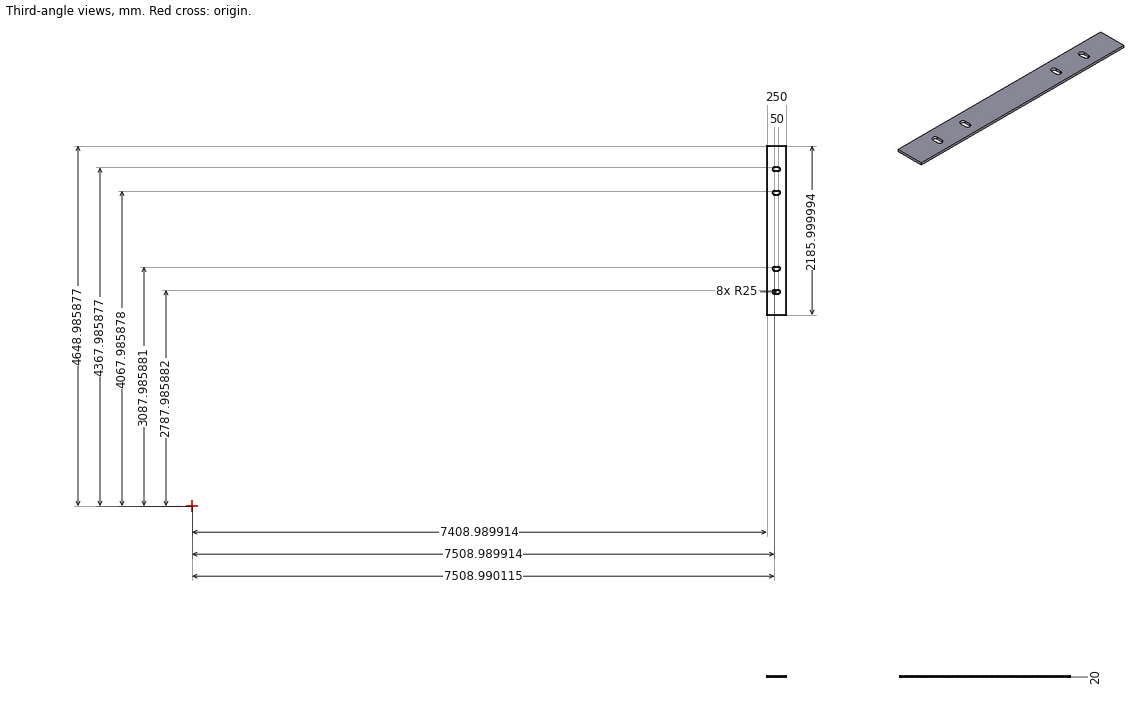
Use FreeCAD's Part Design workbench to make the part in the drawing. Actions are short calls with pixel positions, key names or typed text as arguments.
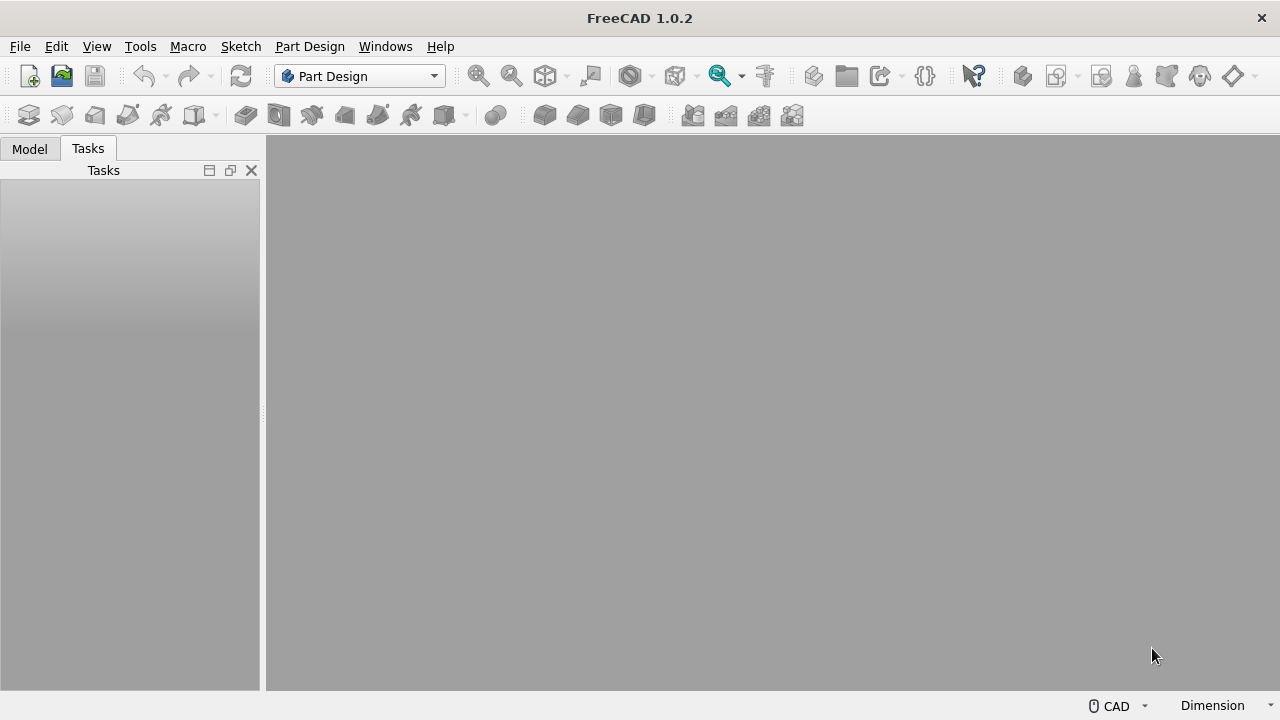
key(ctrl+n)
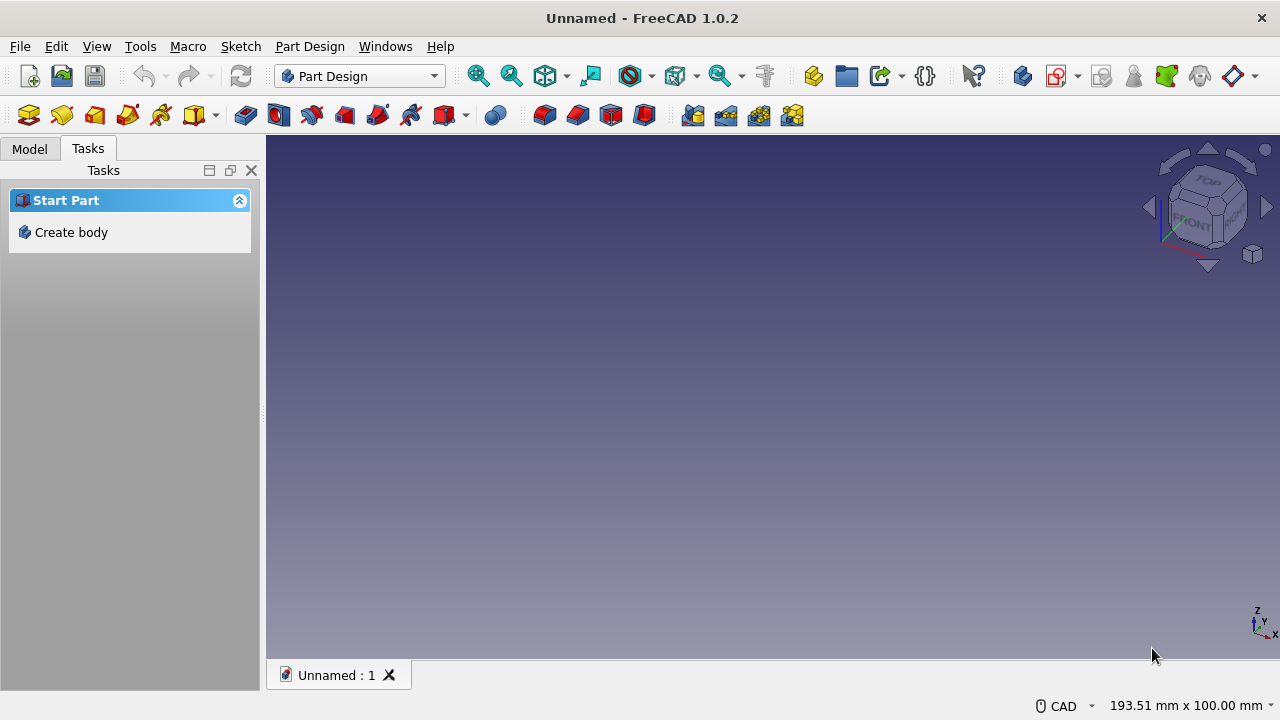
click(1056, 76)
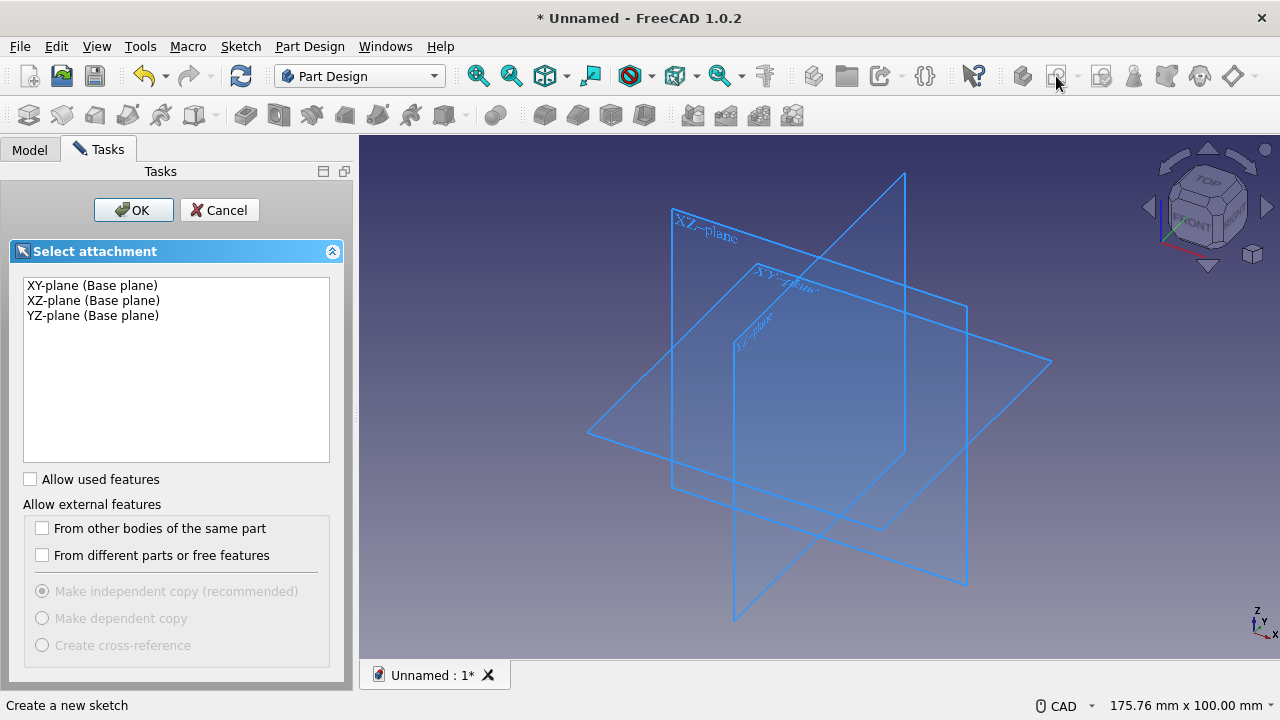
click(84, 286)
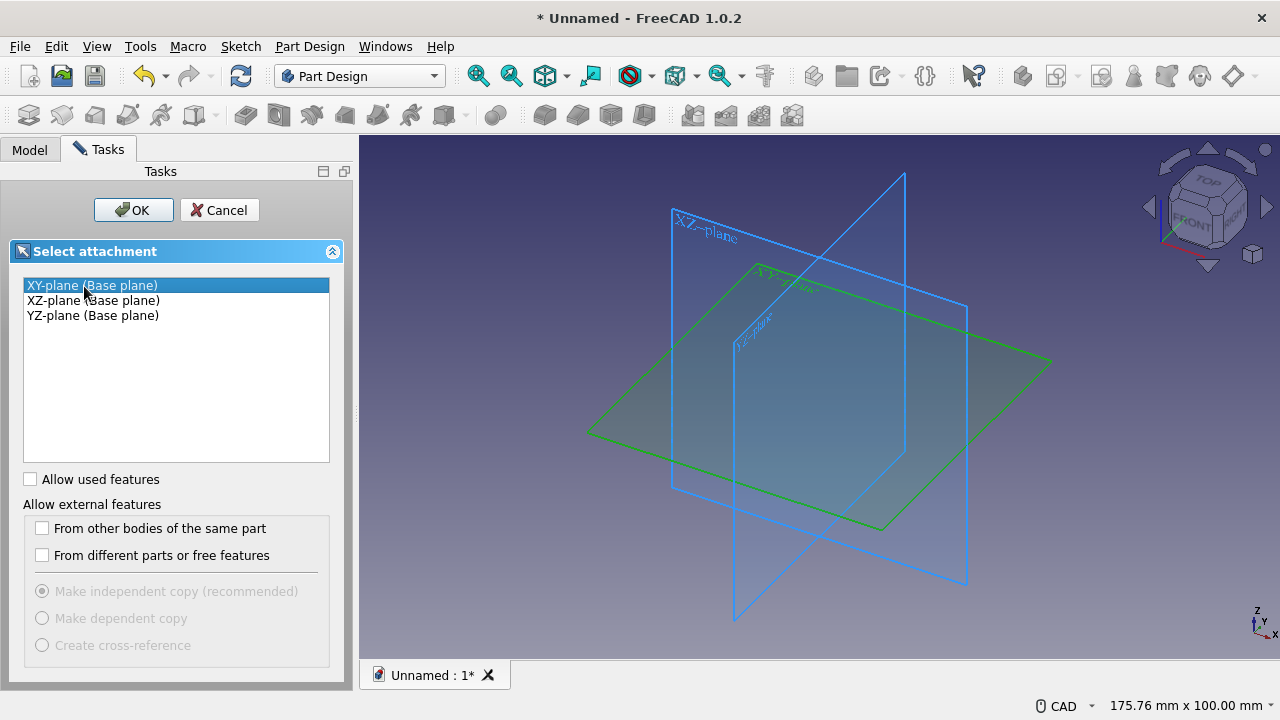
click(134, 210)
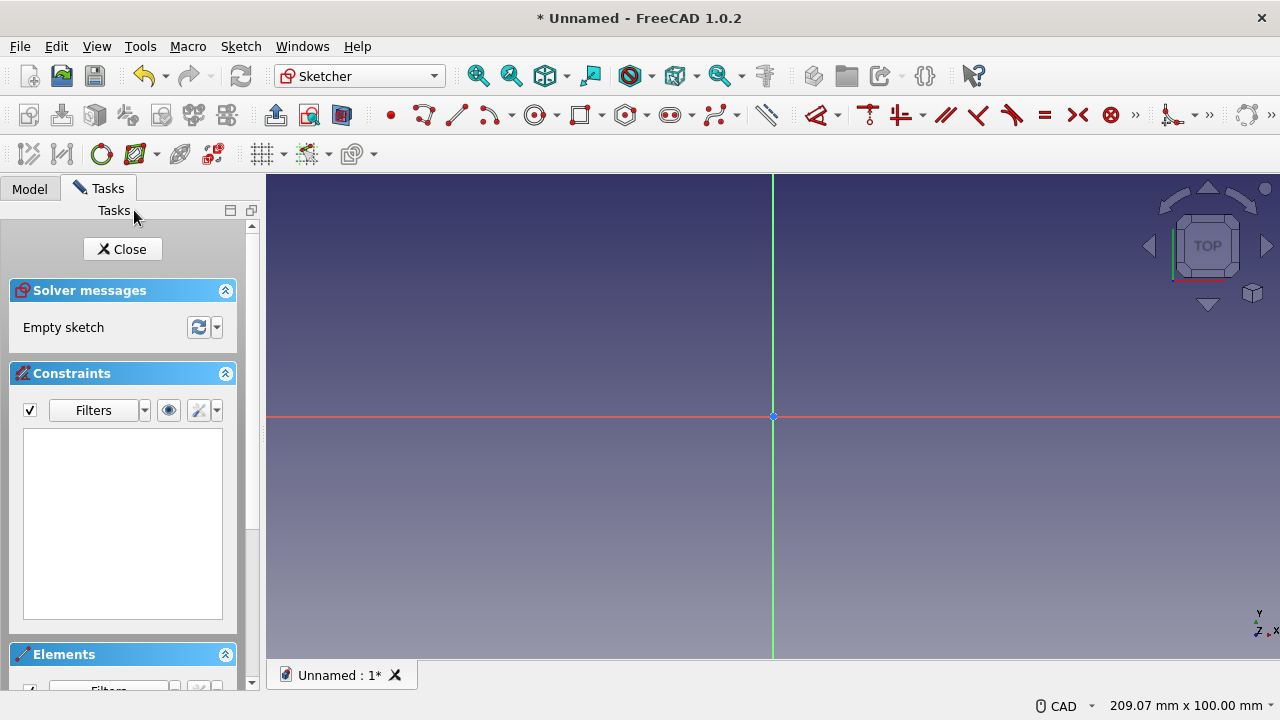
scroll(704, 416, down, 15)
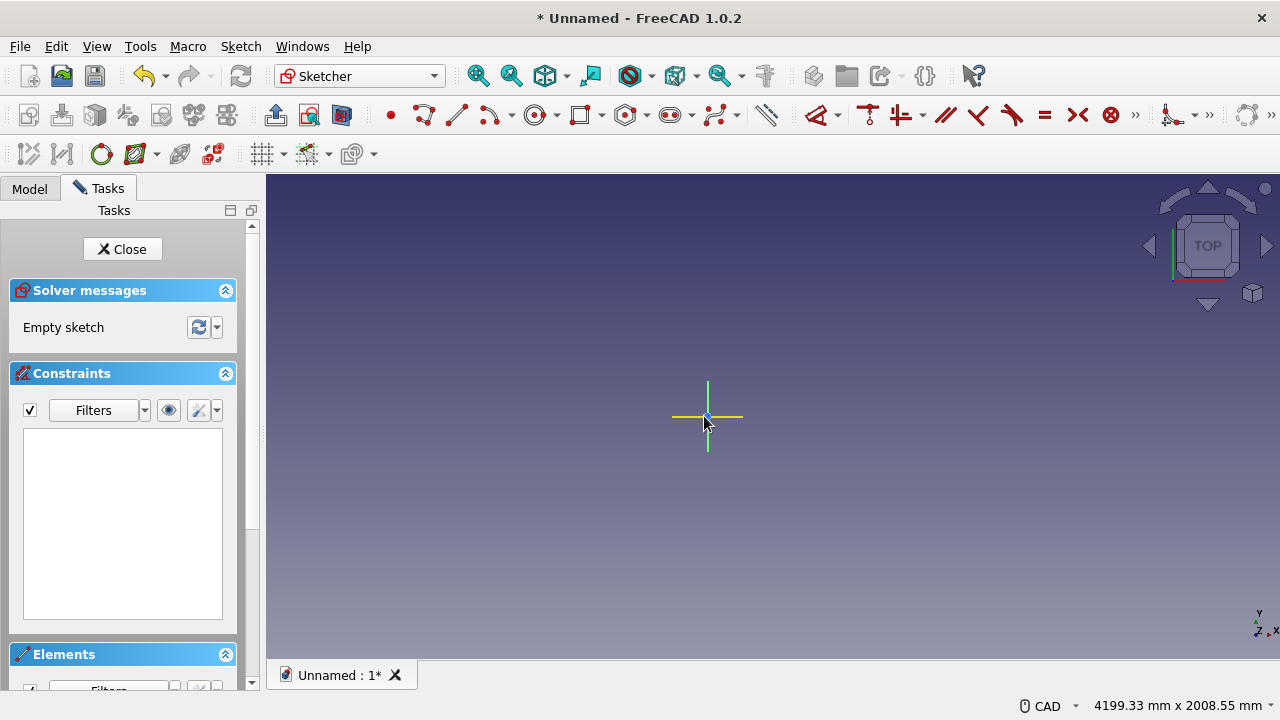
scroll(294, 631, down, 6)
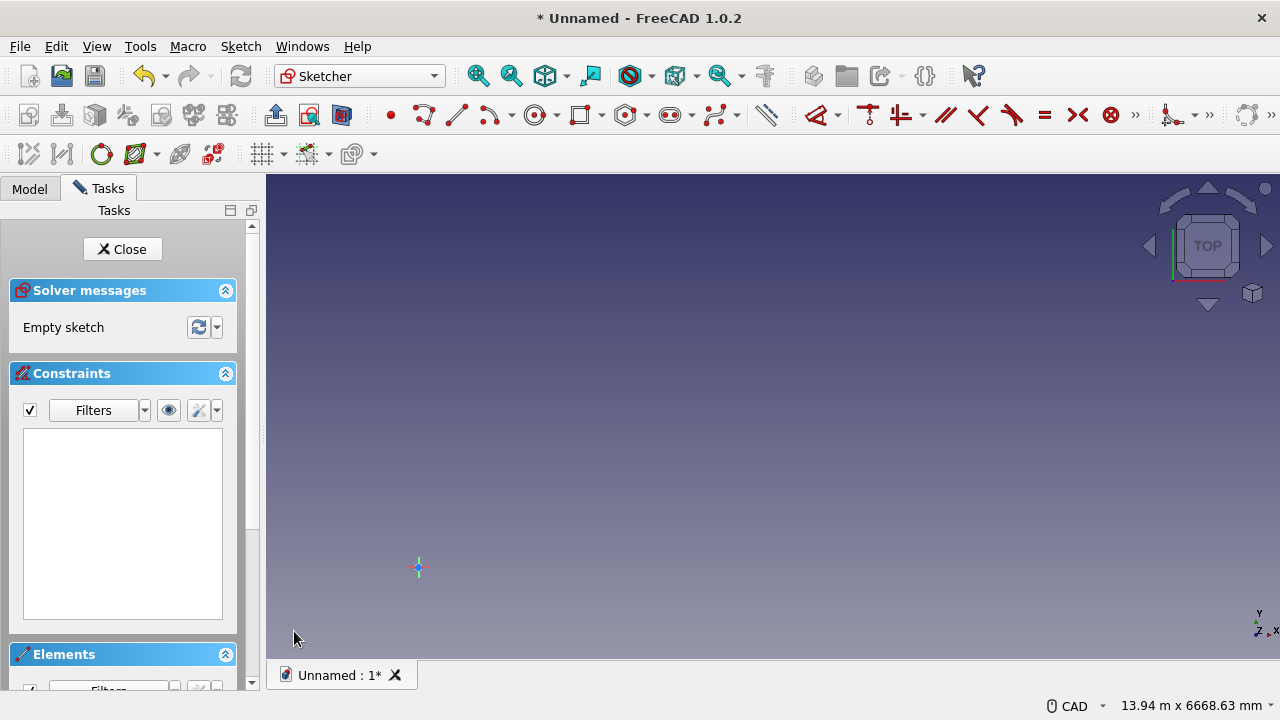
scroll(1115, 202, up, 3)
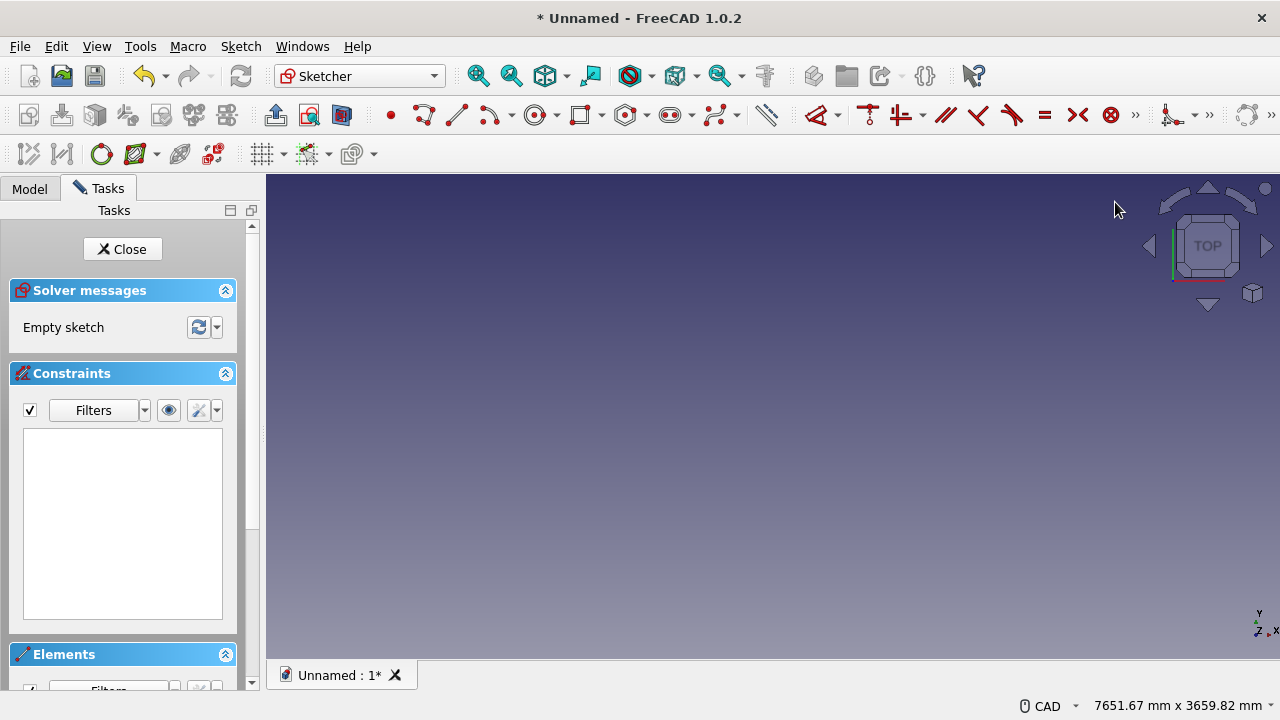
click(580, 116)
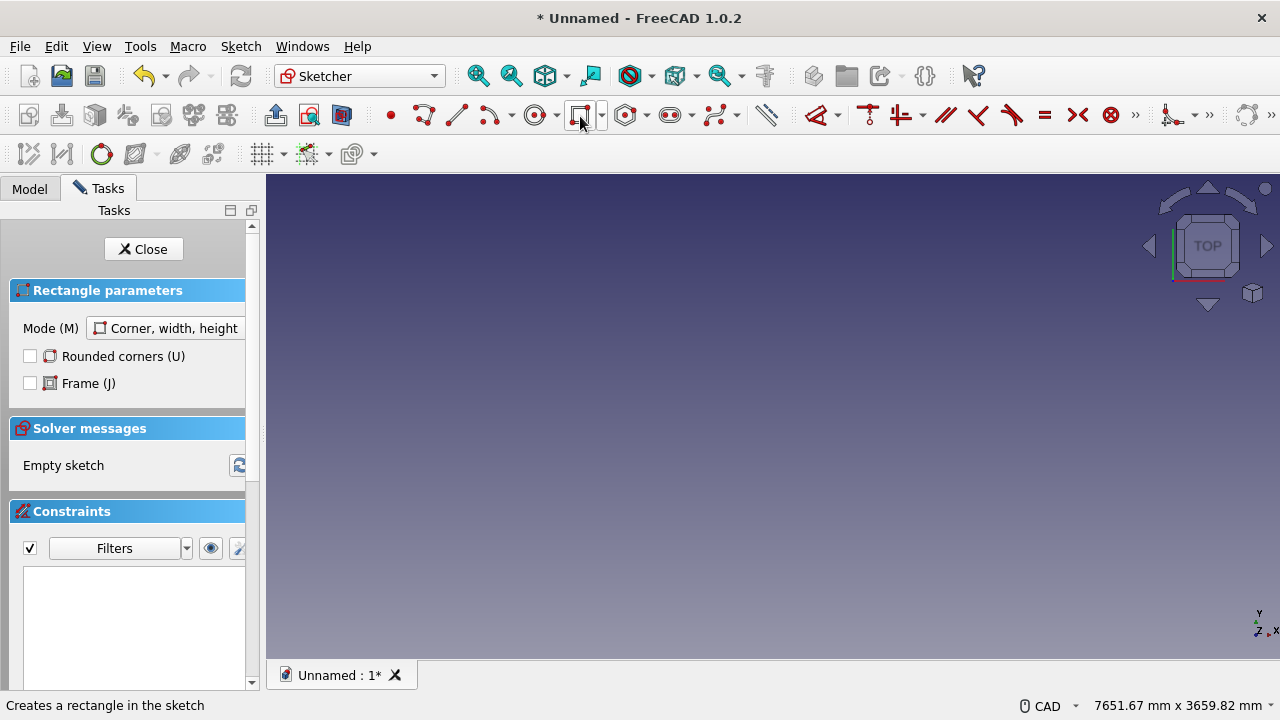
click(827, 251)
click(860, 541)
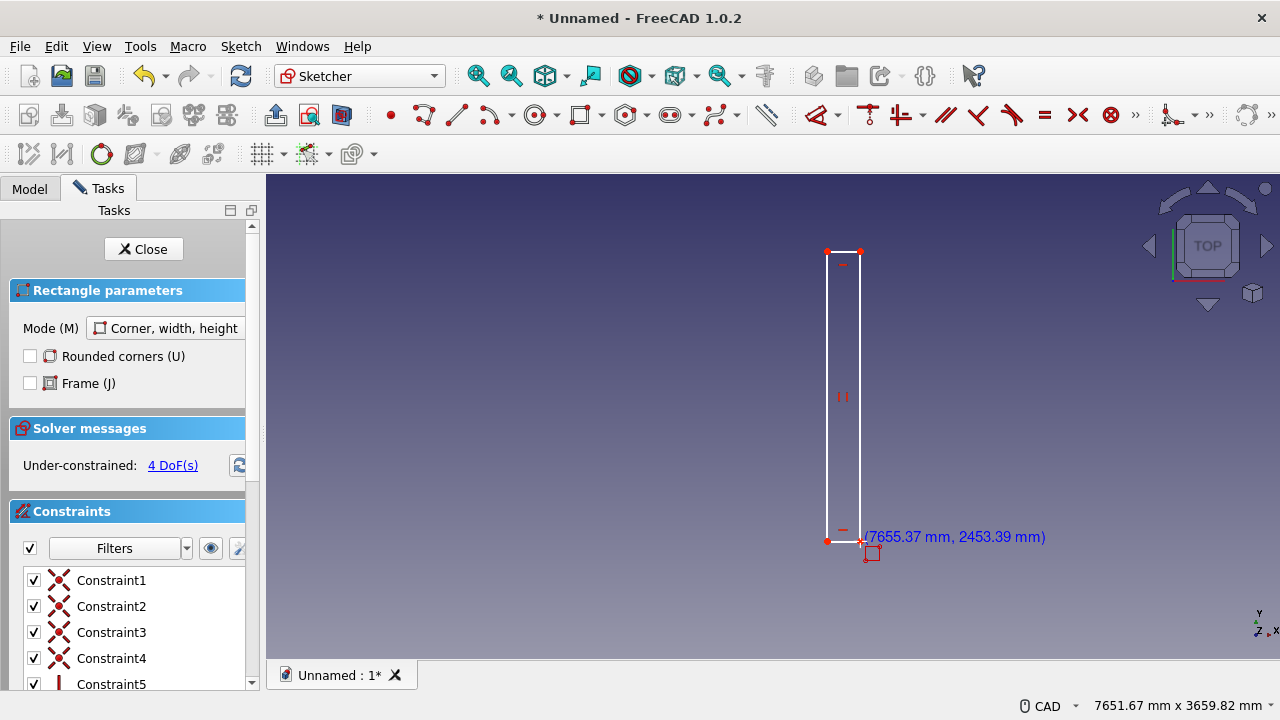
key(g)
key(l)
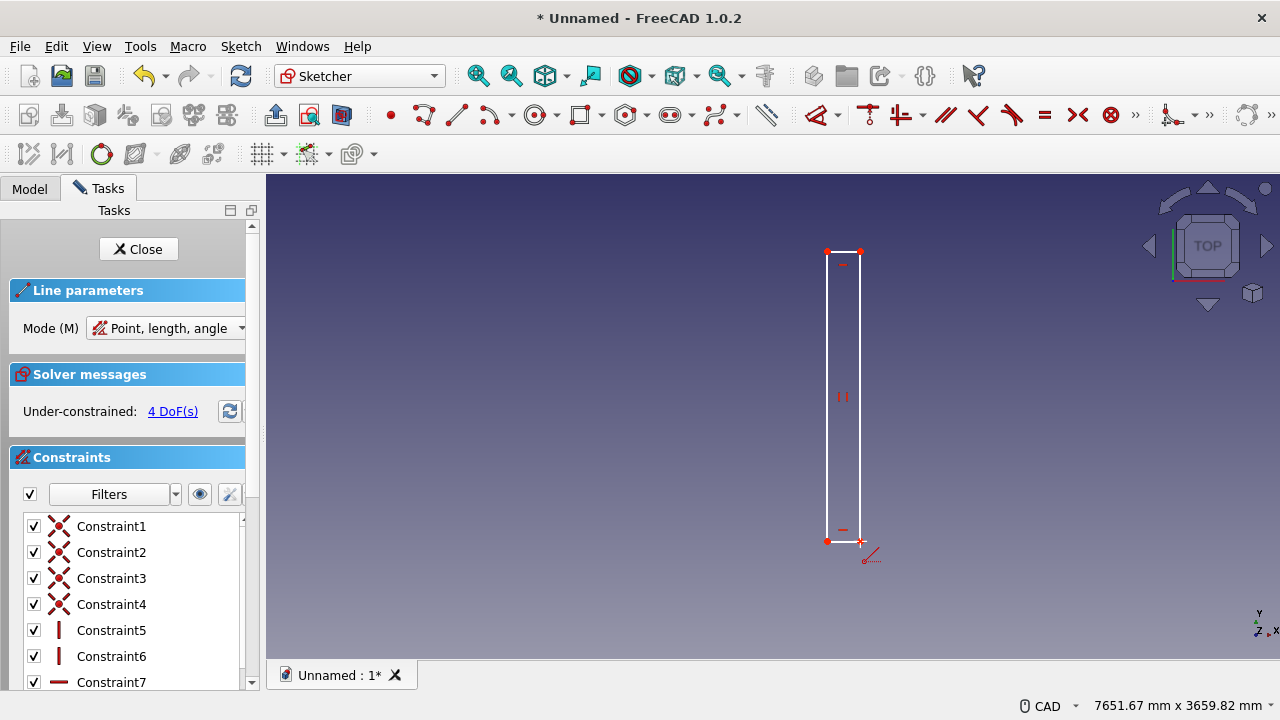
click(841, 498)